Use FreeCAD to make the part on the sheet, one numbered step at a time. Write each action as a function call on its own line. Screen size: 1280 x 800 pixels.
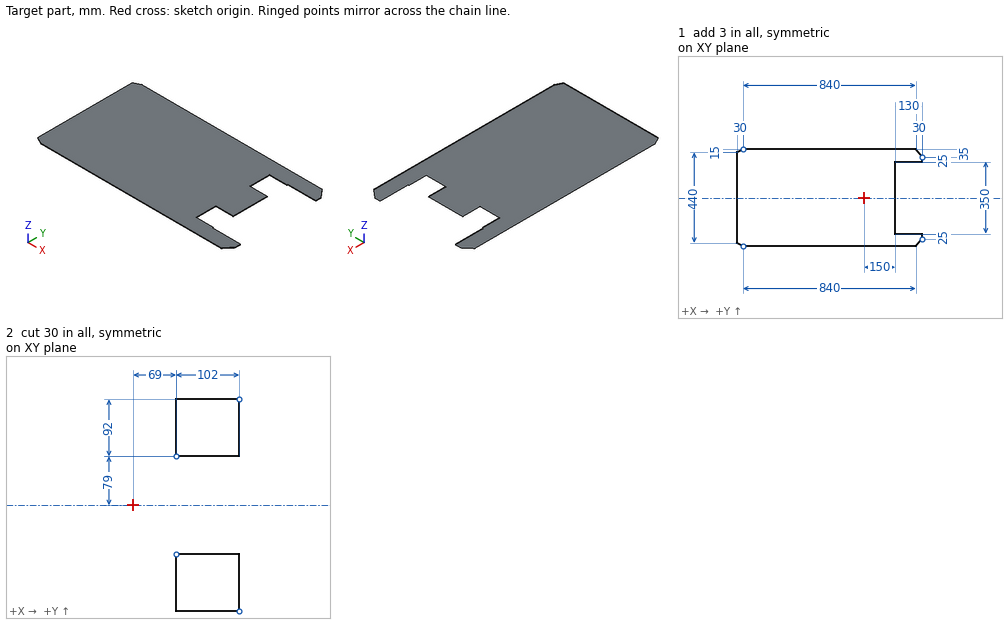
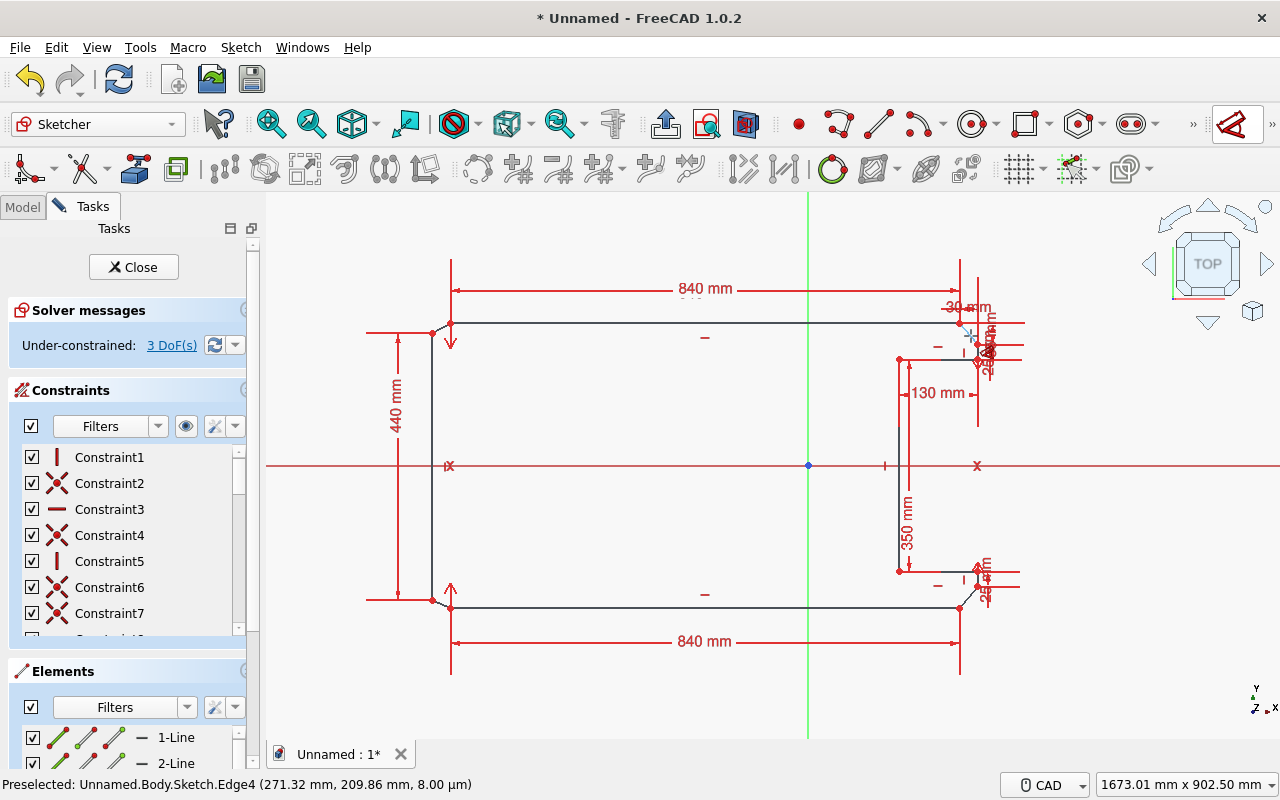
scroll(445, 326, up, 4)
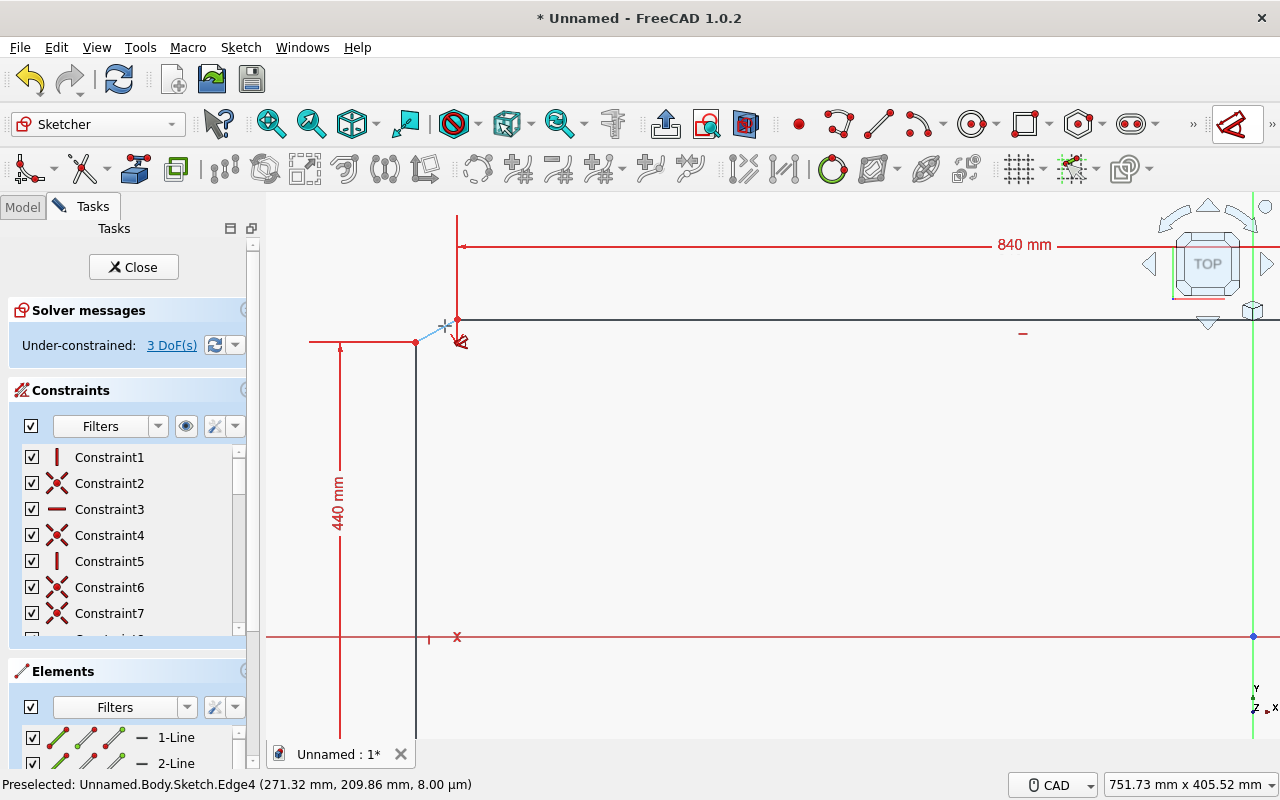
click(445, 327)
click(436, 286)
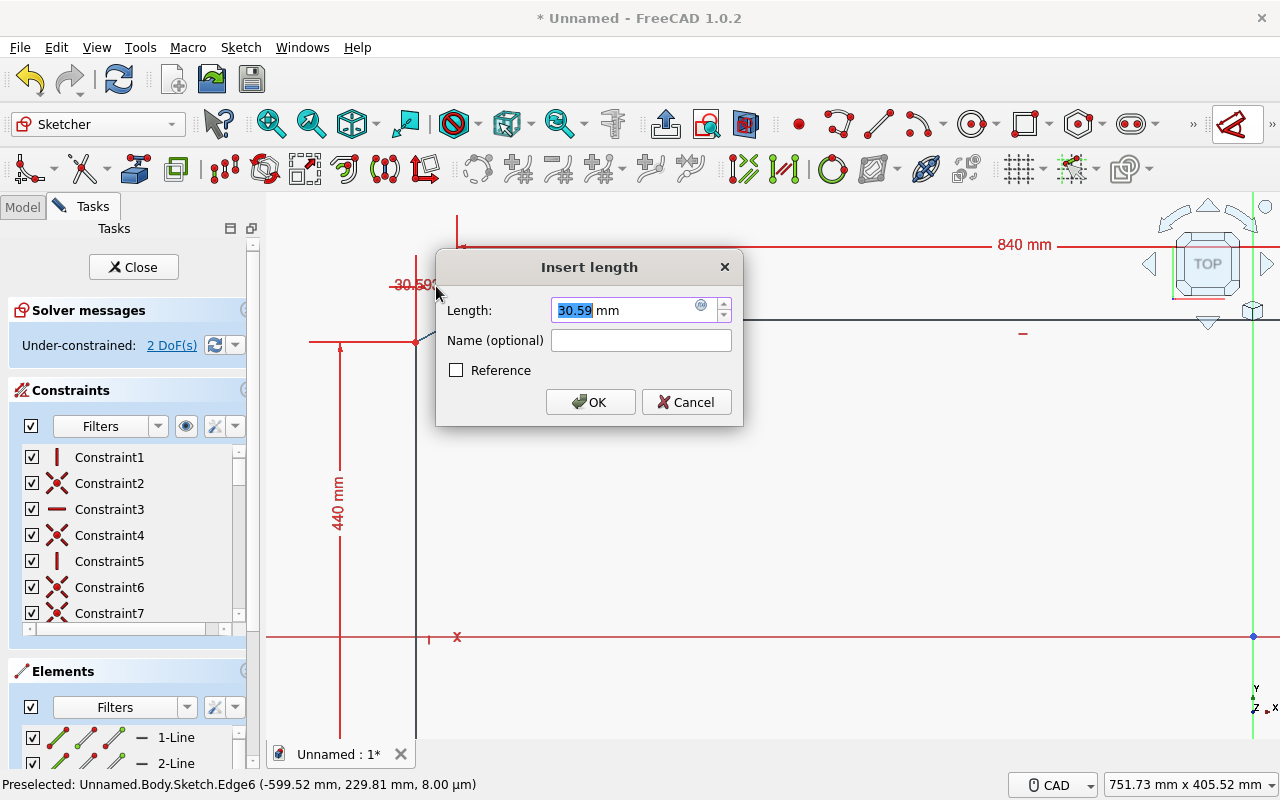
text(30)
key(Return)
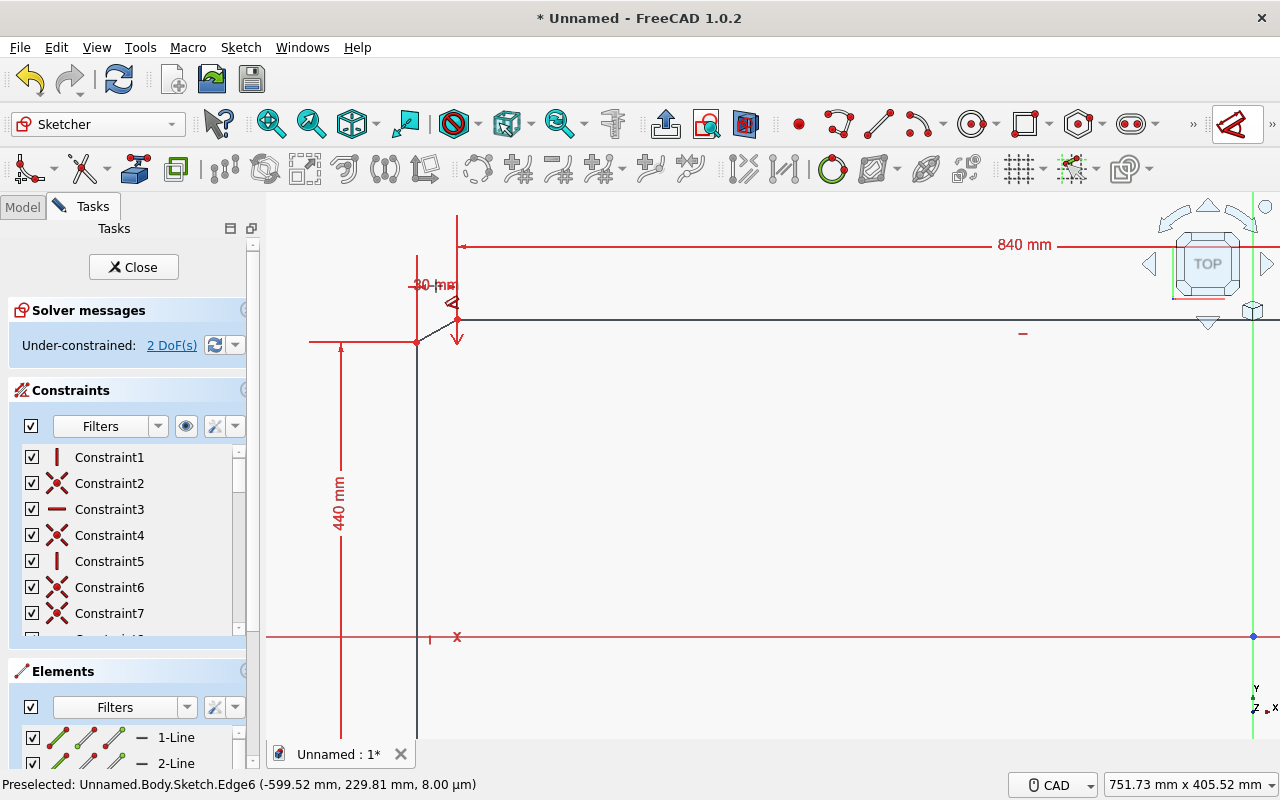
scroll(445, 327, up, 4)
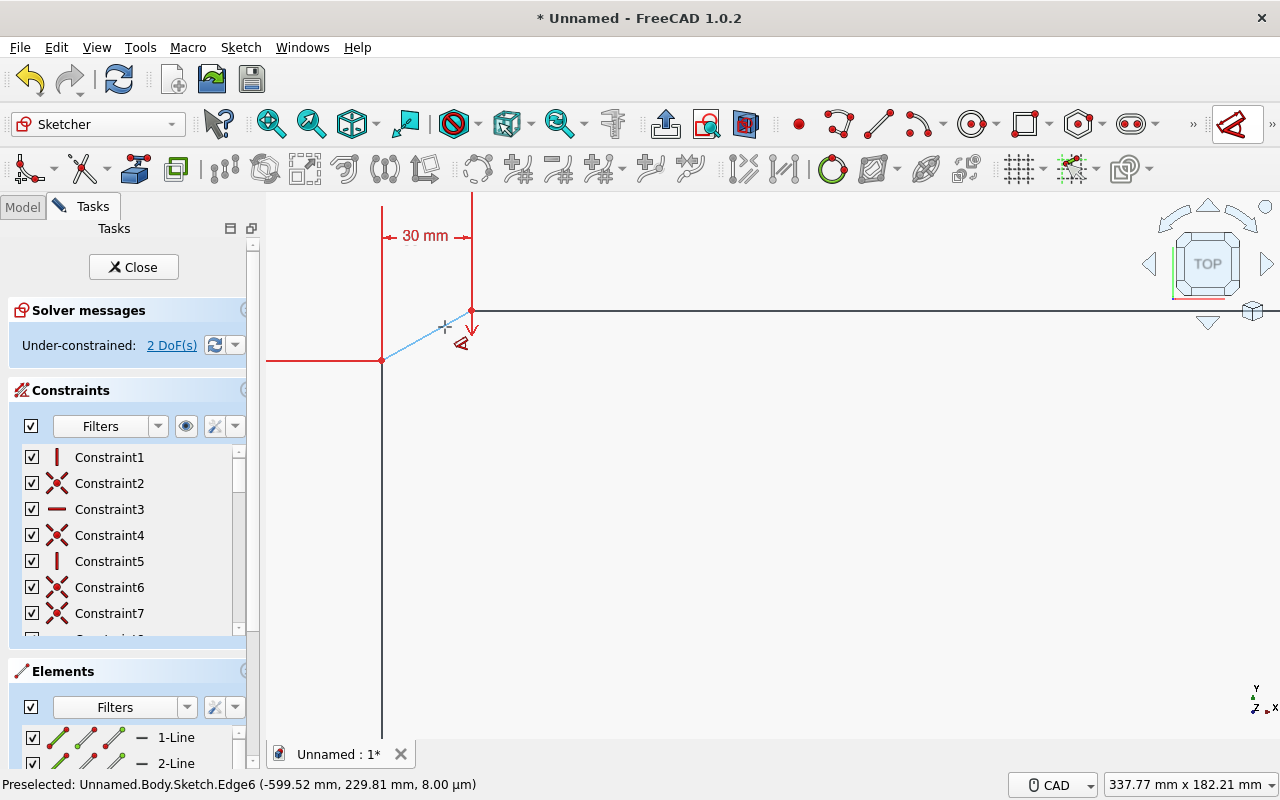
click(445, 326)
click(348, 336)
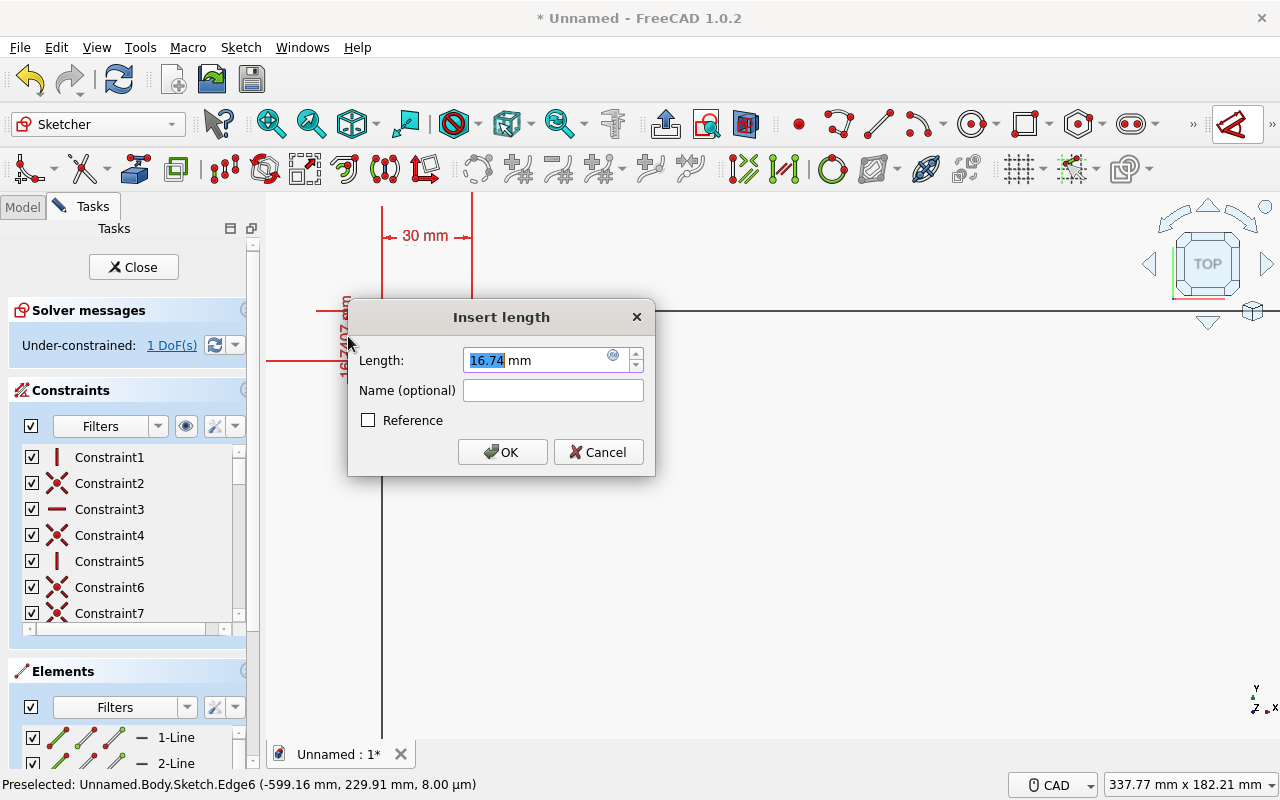
text(15)
key(Return)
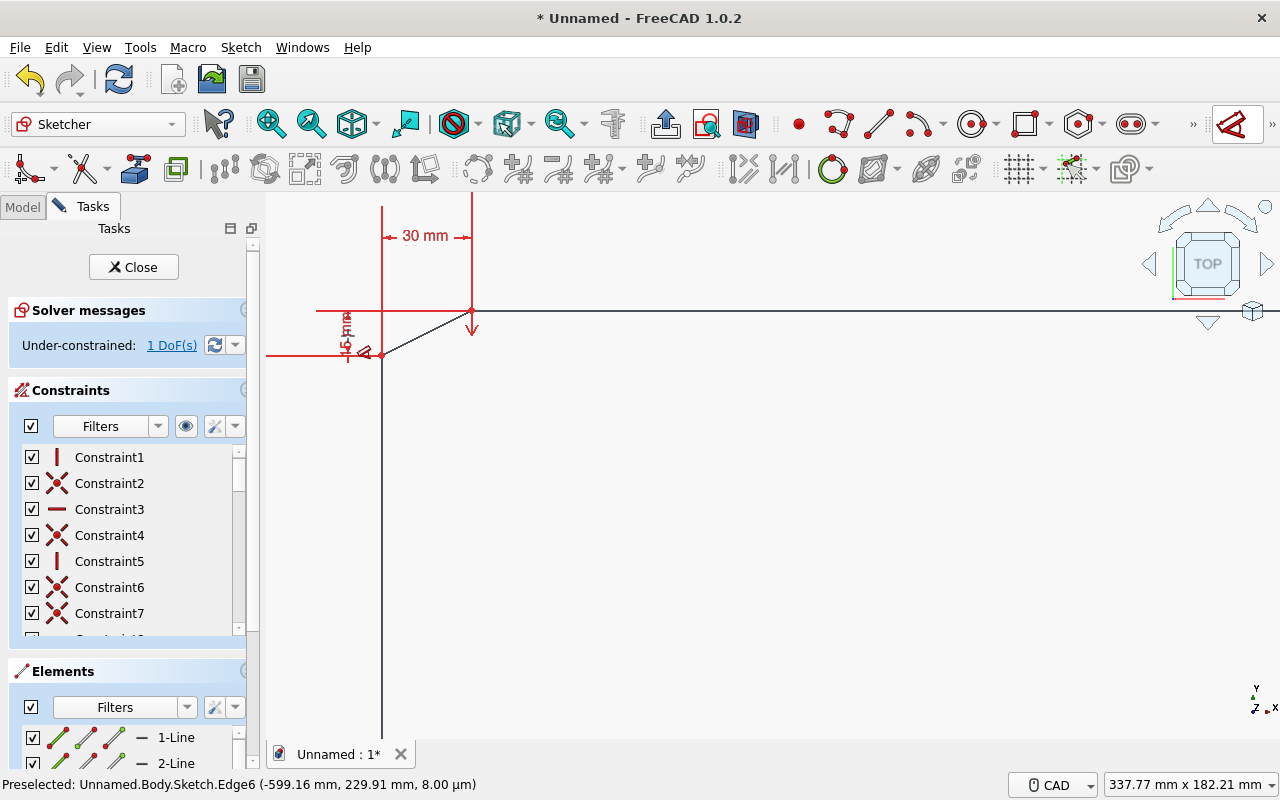
scroll(444, 326, down, 8)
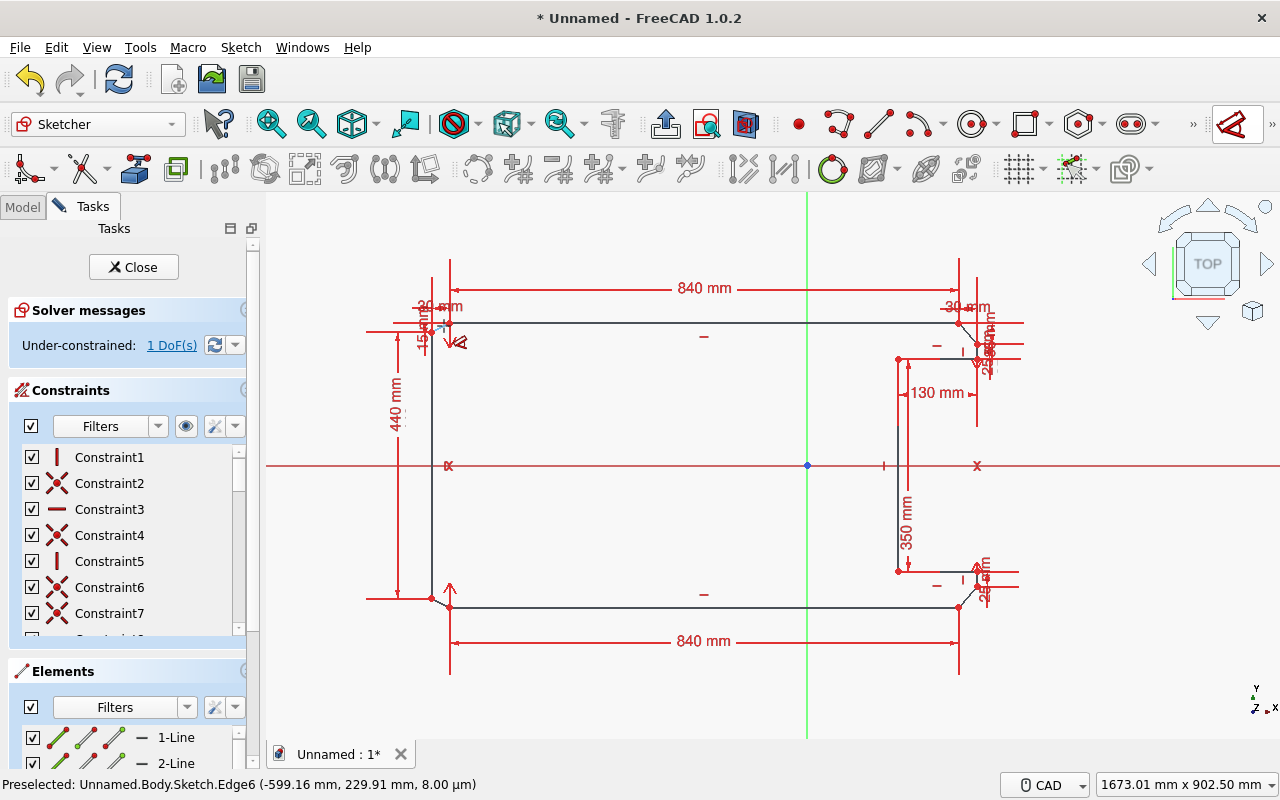
click(898, 572)
click(853, 432)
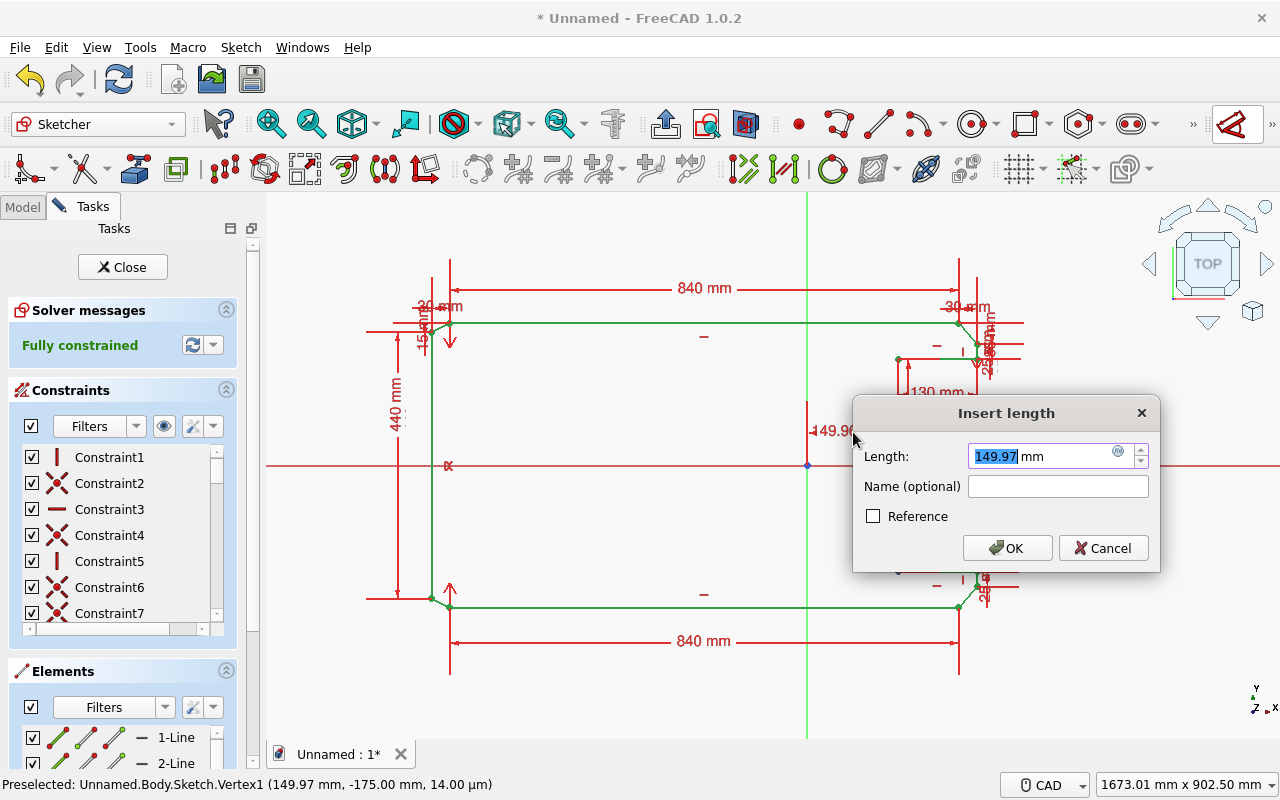
text(150)
key(Return)
key(Escape)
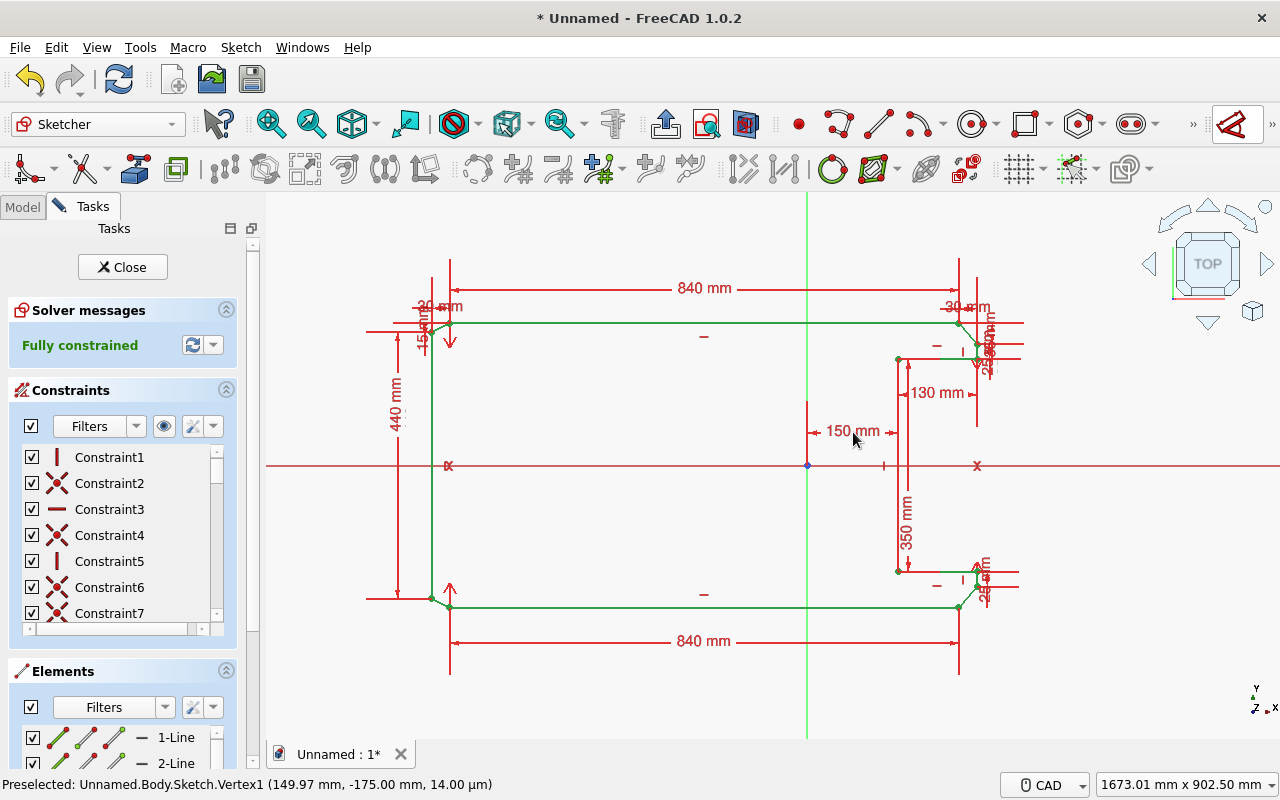
click(123, 267)